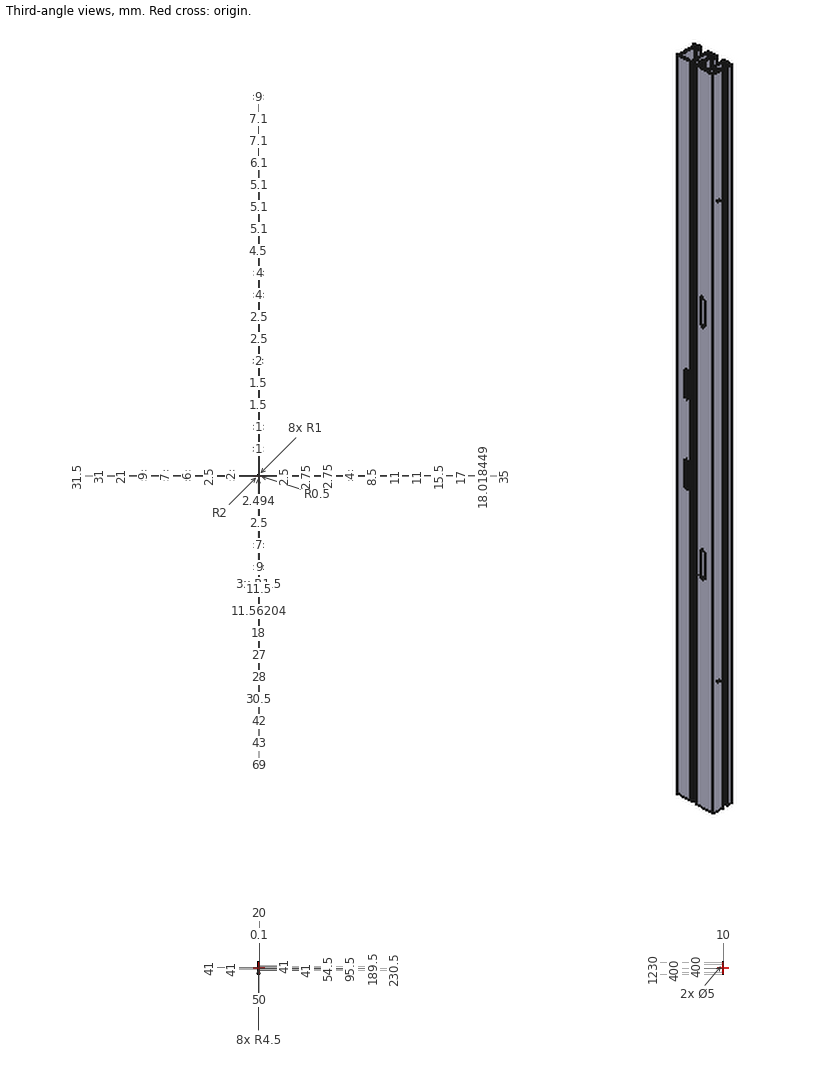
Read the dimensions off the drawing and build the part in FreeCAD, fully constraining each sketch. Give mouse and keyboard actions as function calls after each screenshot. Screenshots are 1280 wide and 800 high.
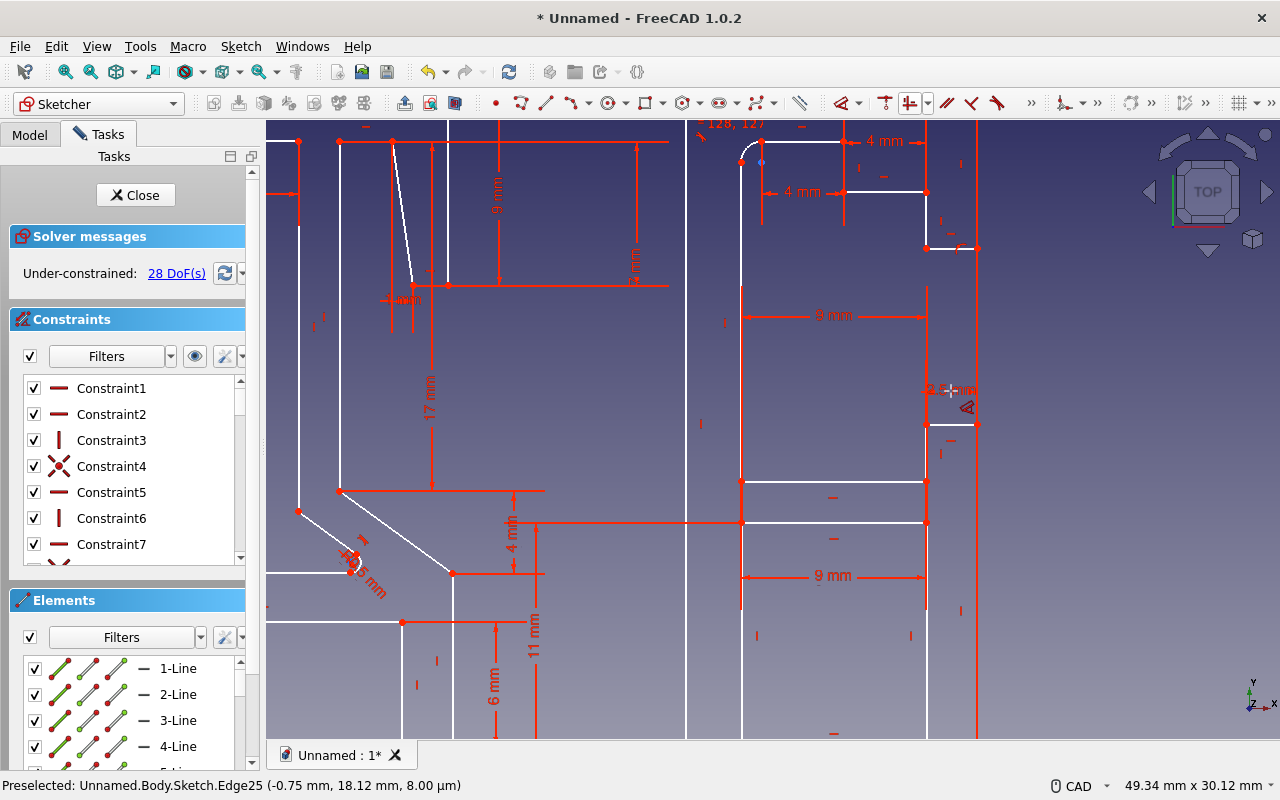
click(844, 157)
click(878, 170)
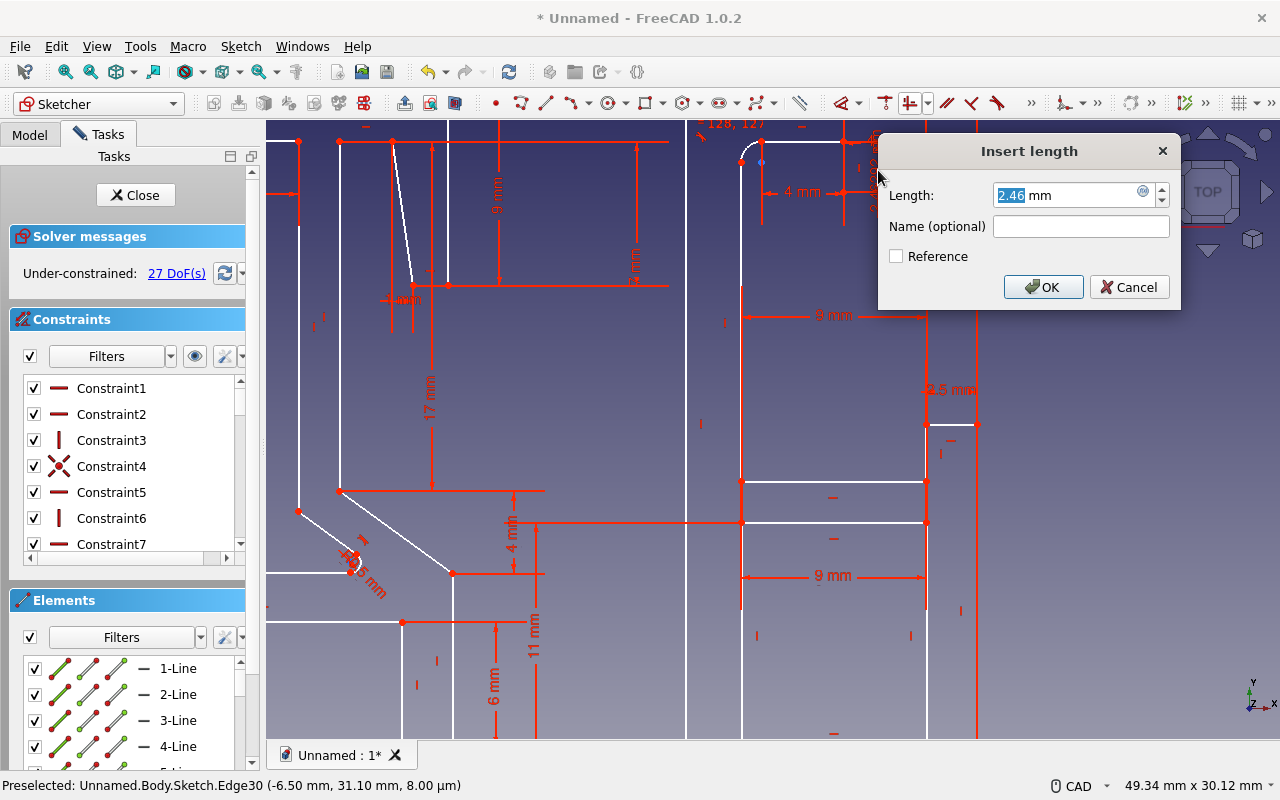
text(2.5)
key(Return)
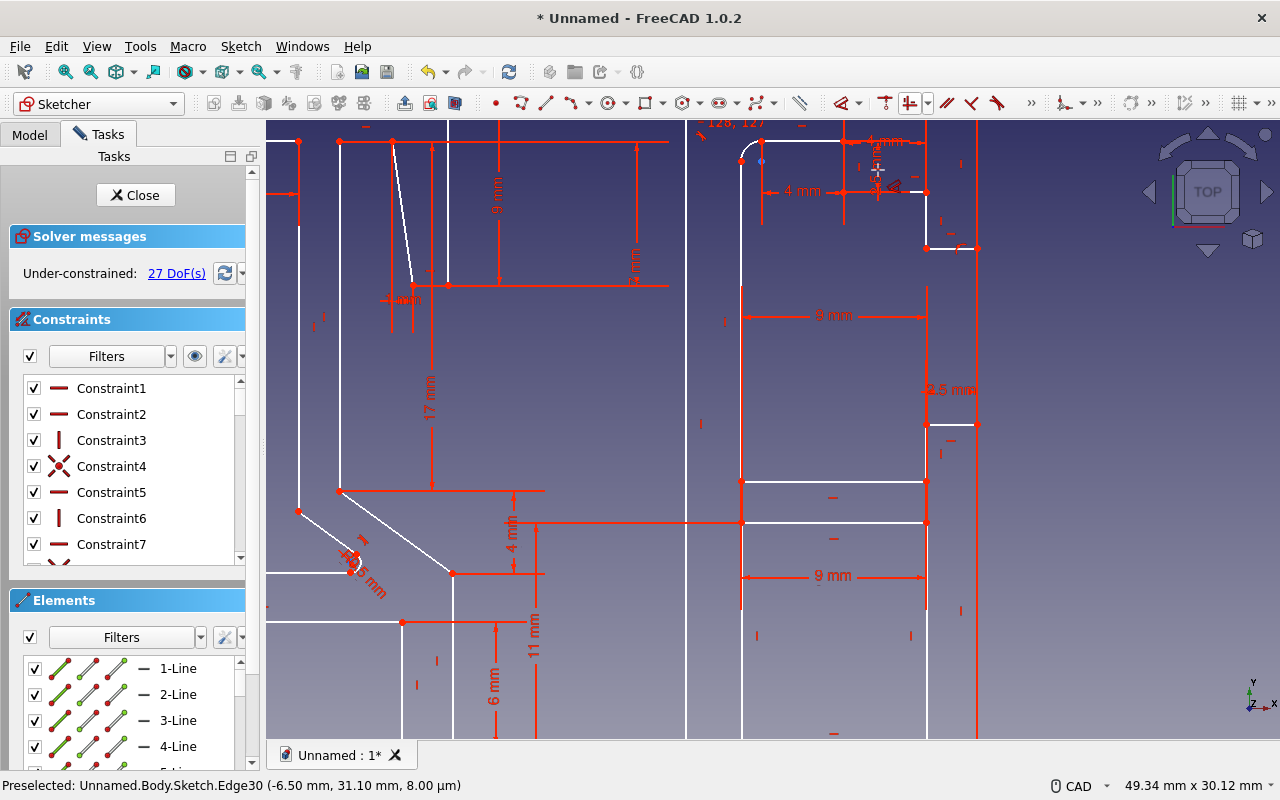
scroll(964, 425, down, 5)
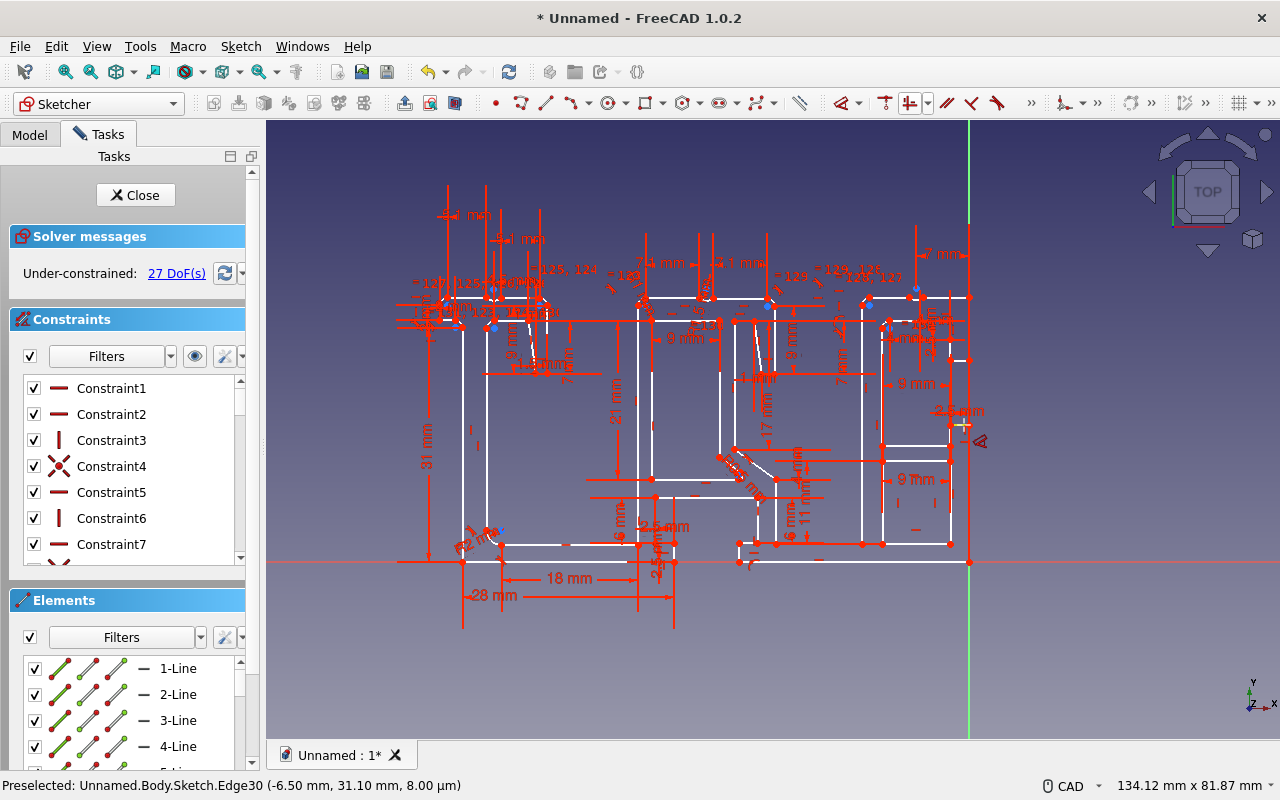
click(955, 298)
click(946, 216)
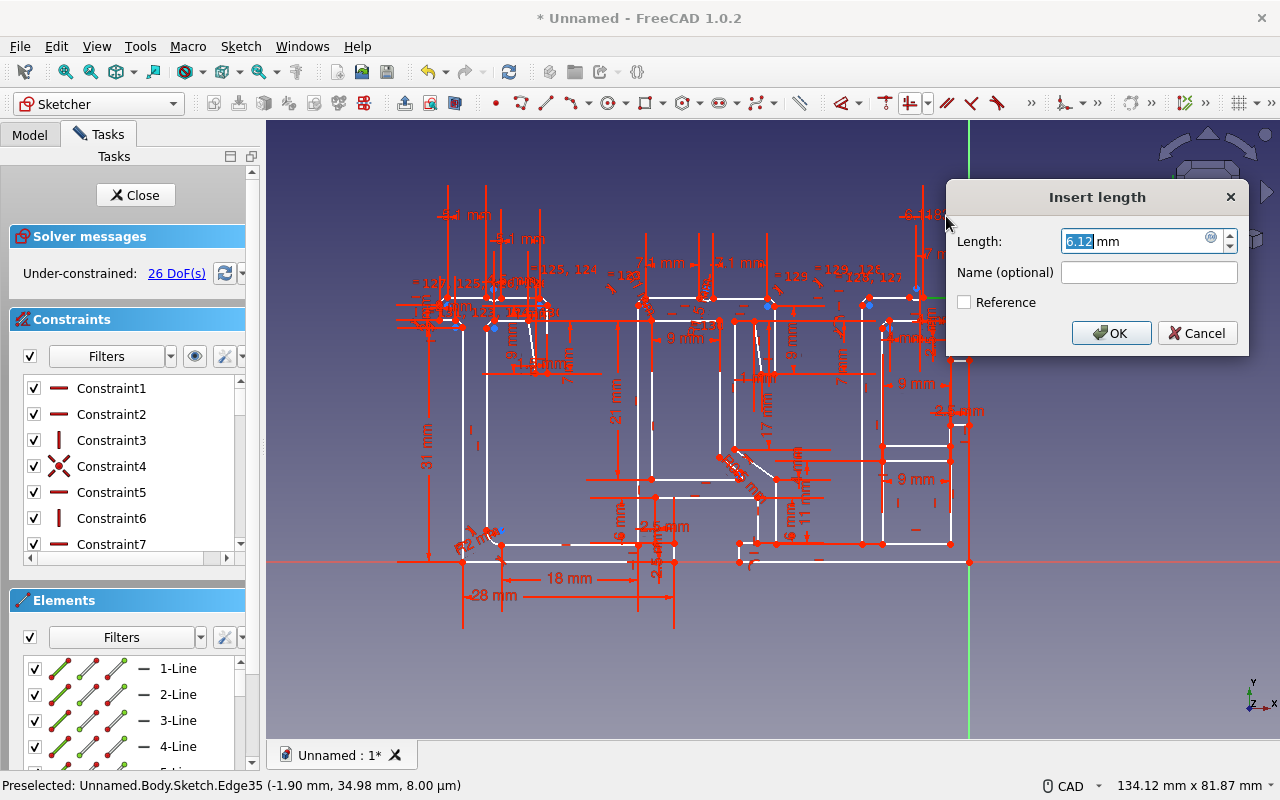
text(6.1)
key(Return)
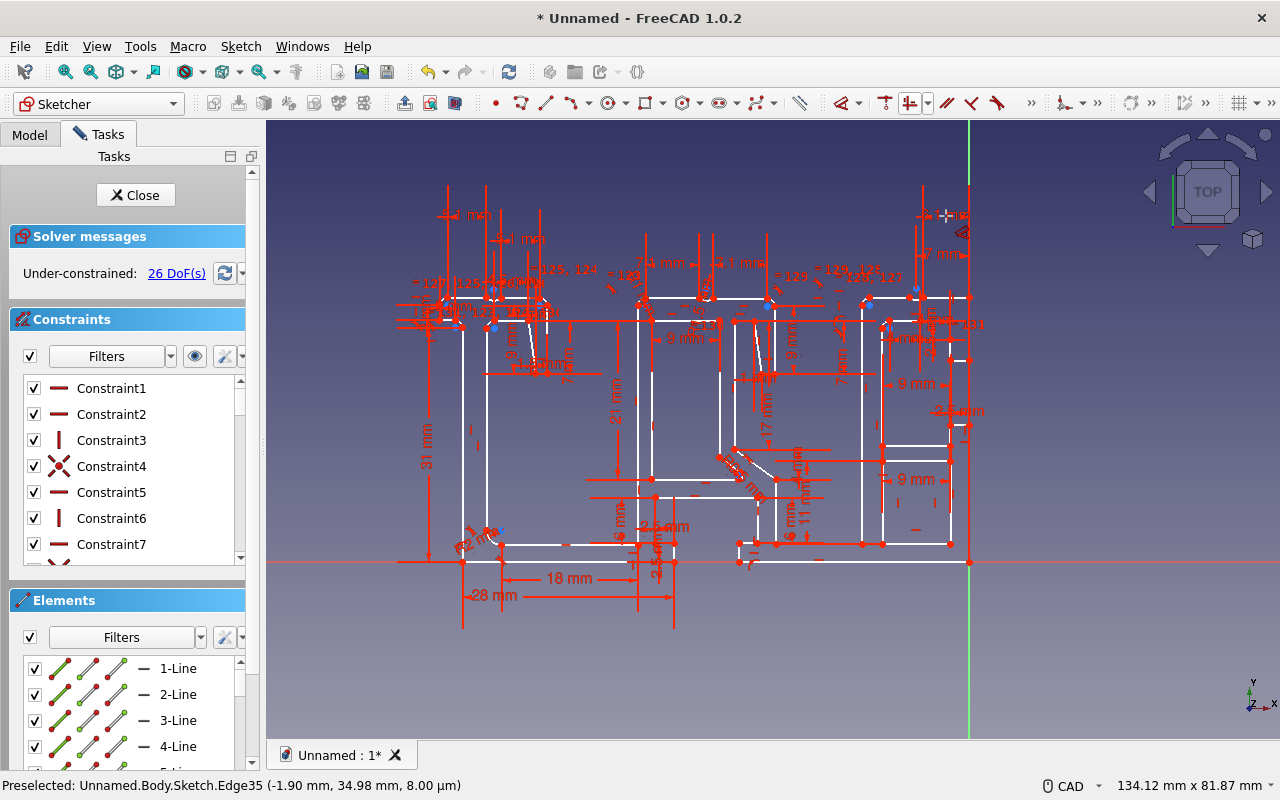
click(898, 298)
click(876, 216)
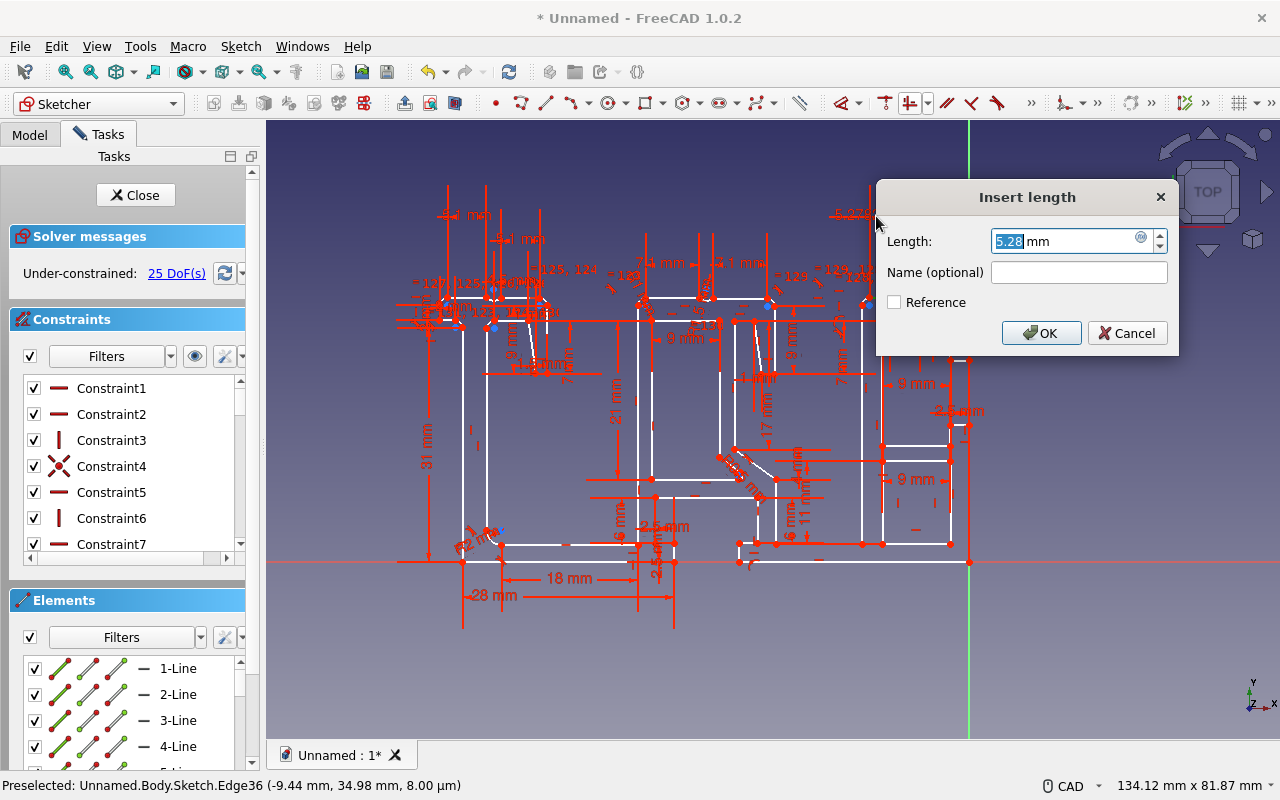
text(5.1)
key(Return)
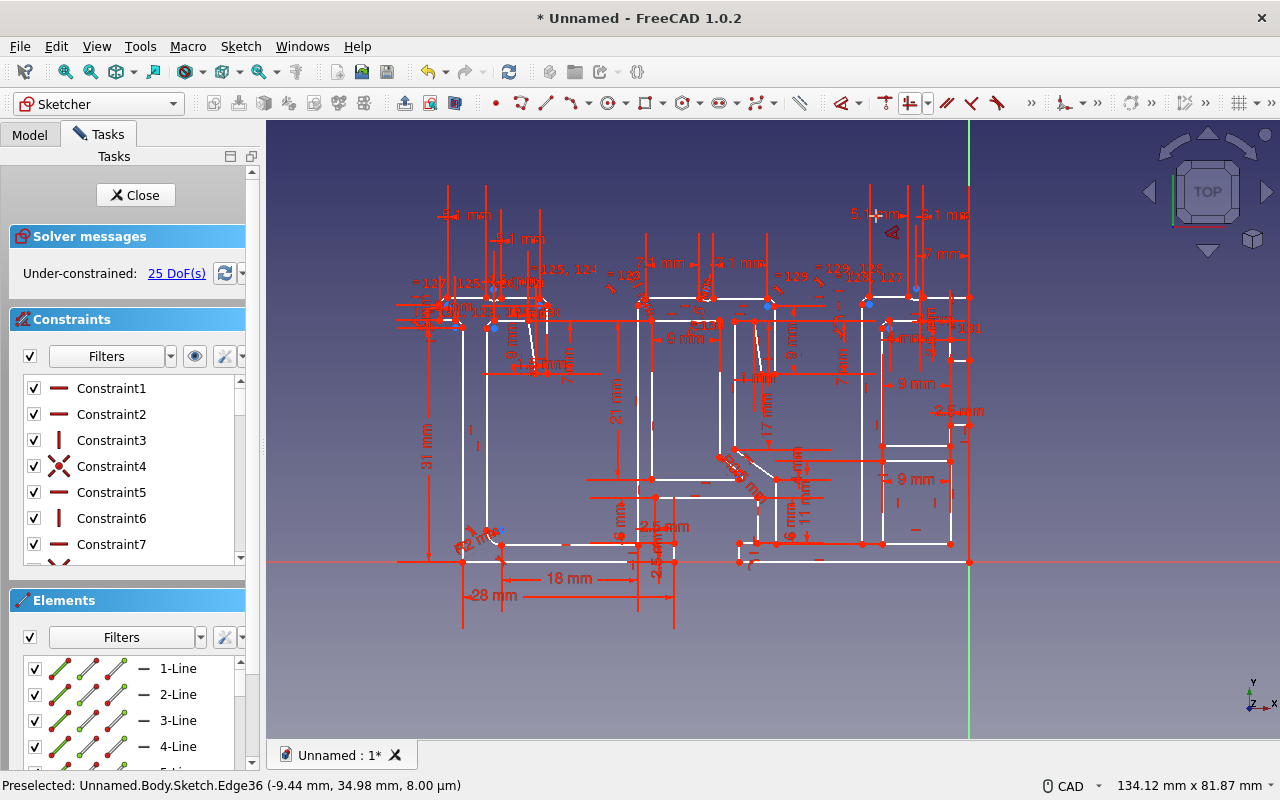
click(776, 525)
click(834, 497)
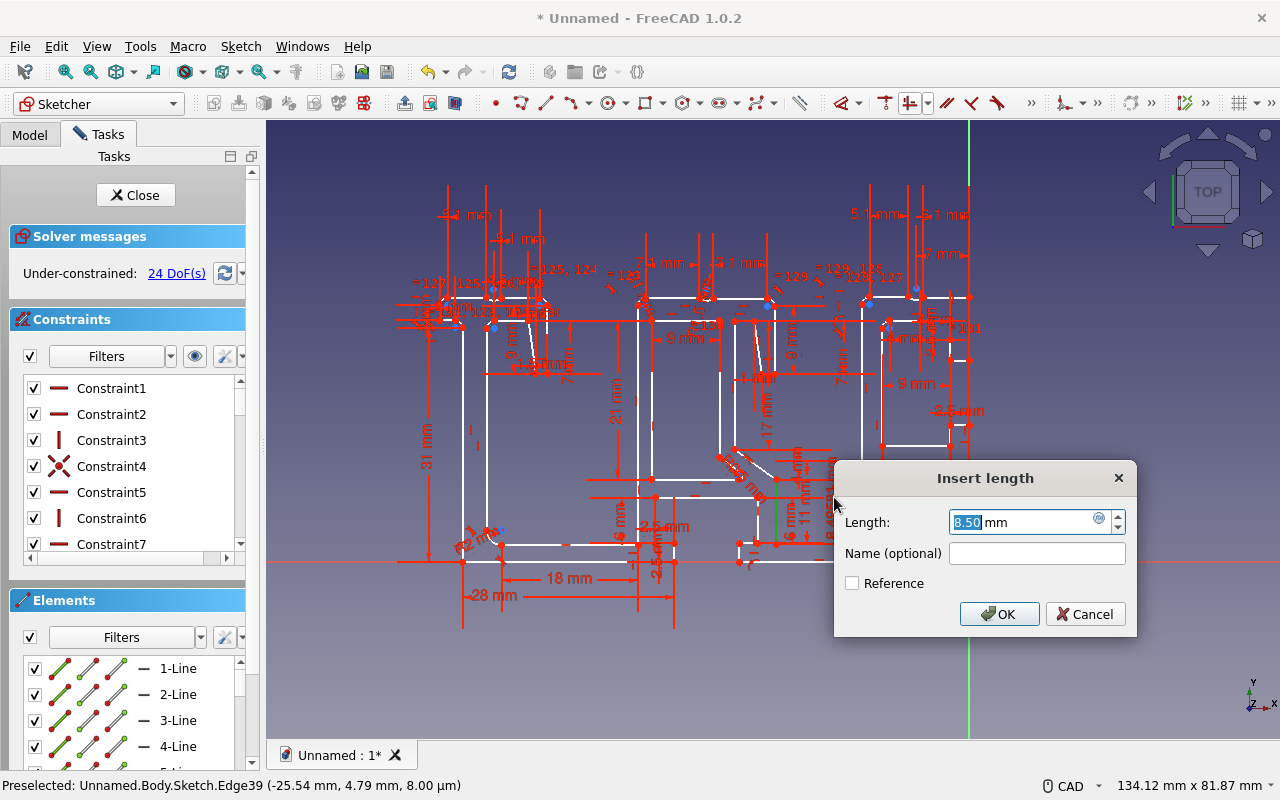
text(8.5)
key(Return)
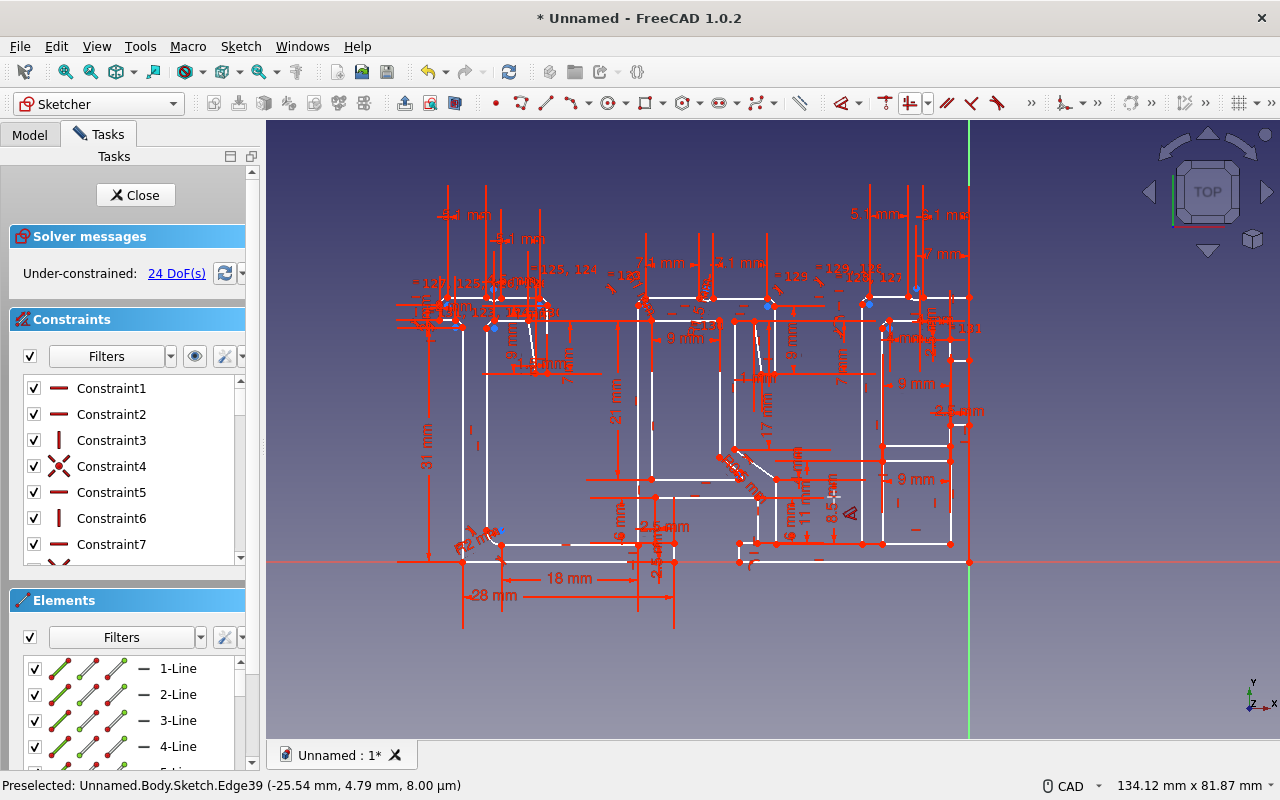
scroll(744, 321, up, 4)